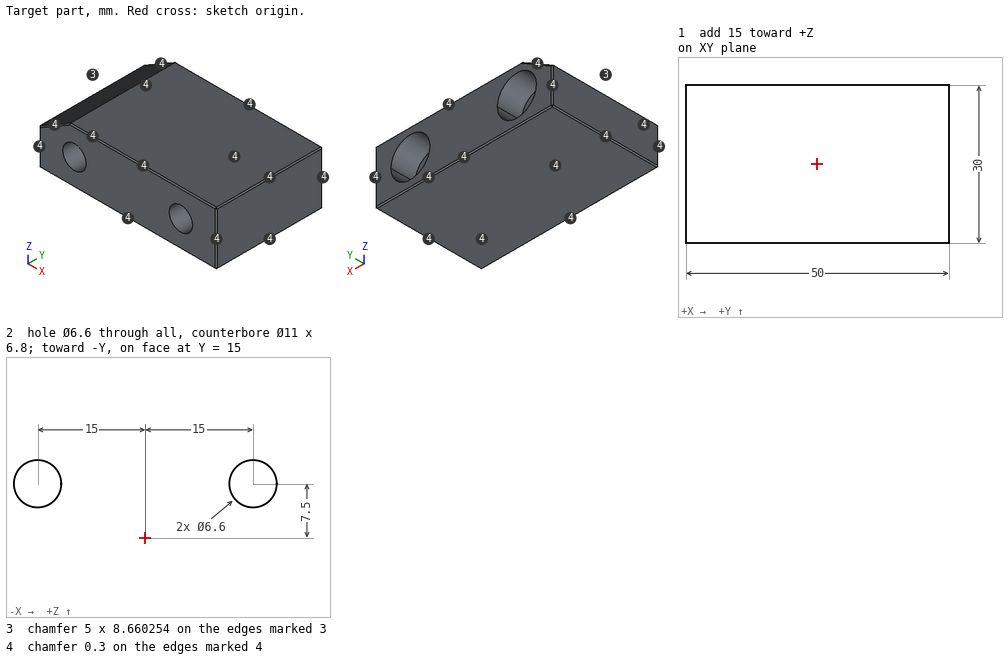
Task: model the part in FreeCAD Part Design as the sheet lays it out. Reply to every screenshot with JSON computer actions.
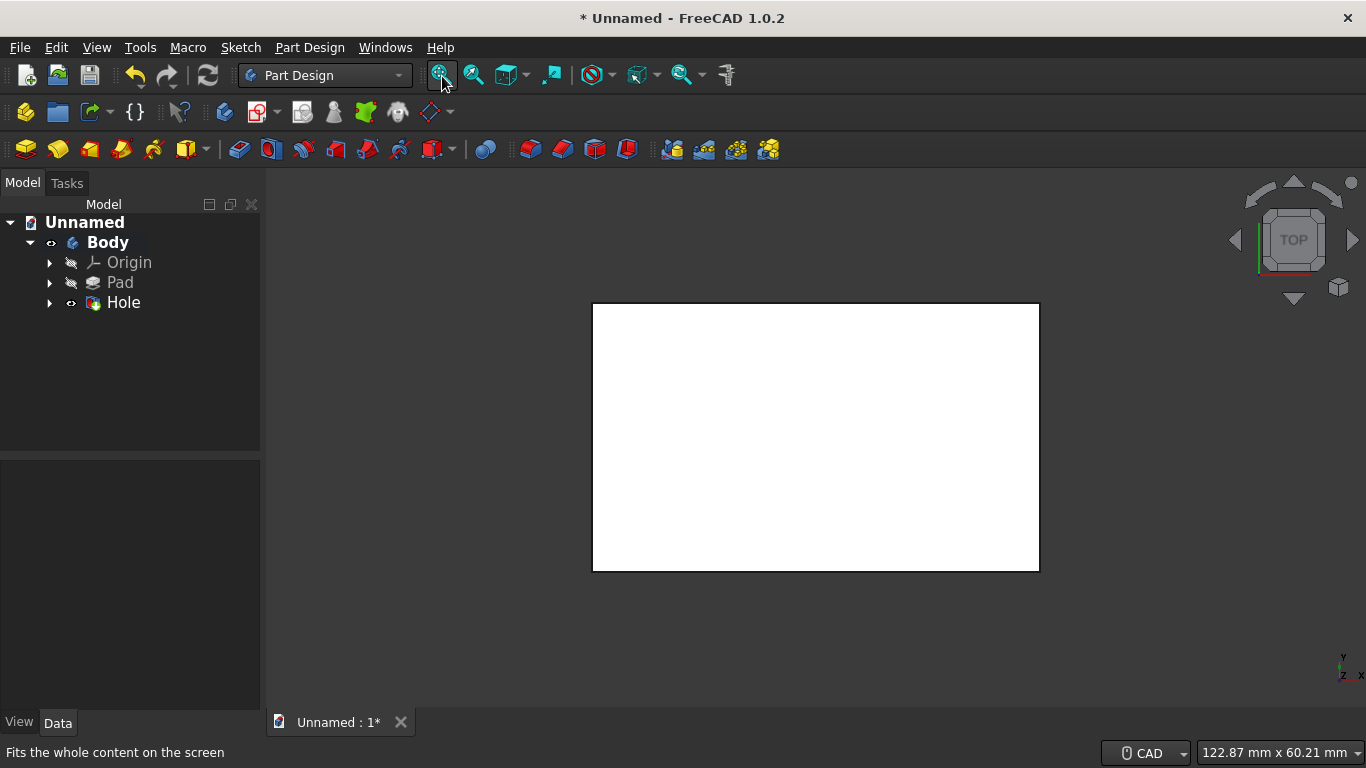
{"action": "left_click", "coordinate": [592, 437]}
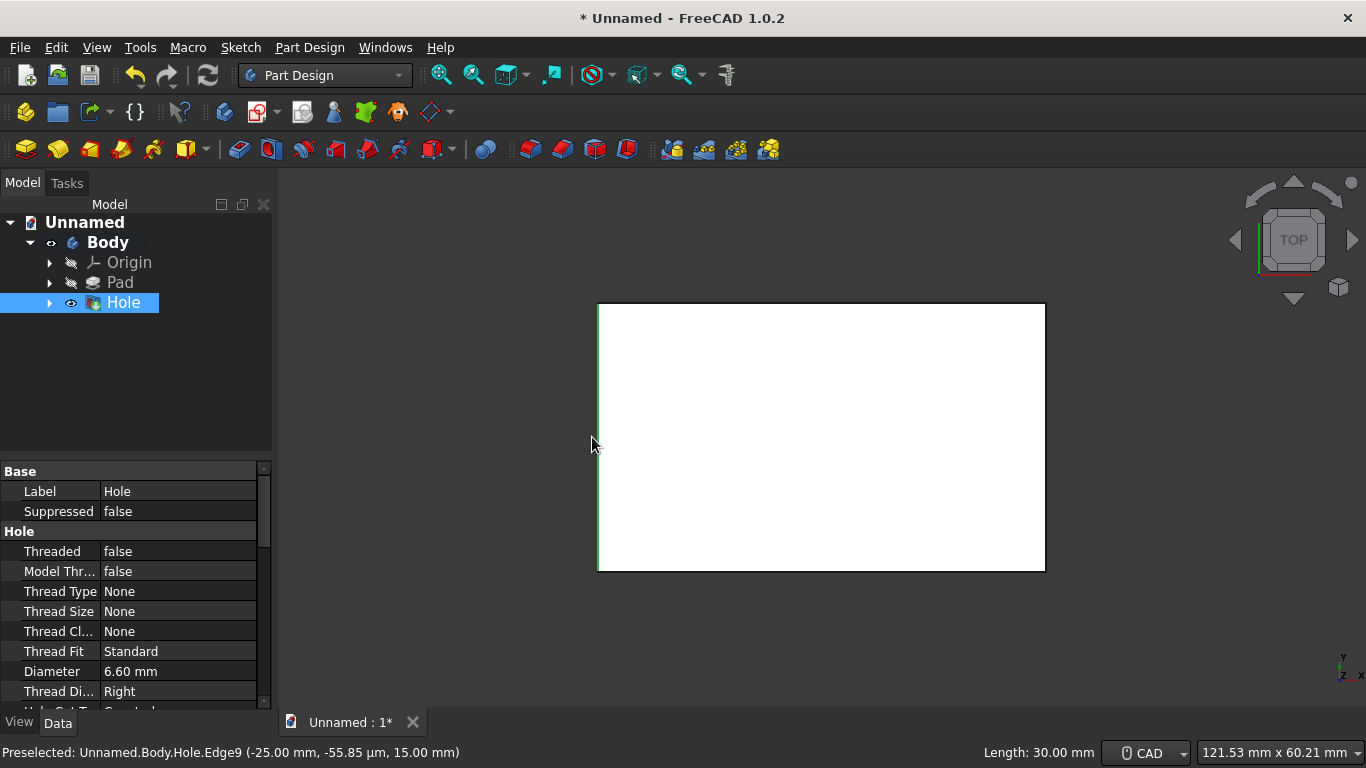
{"action": "left_click", "coordinate": [564, 150]}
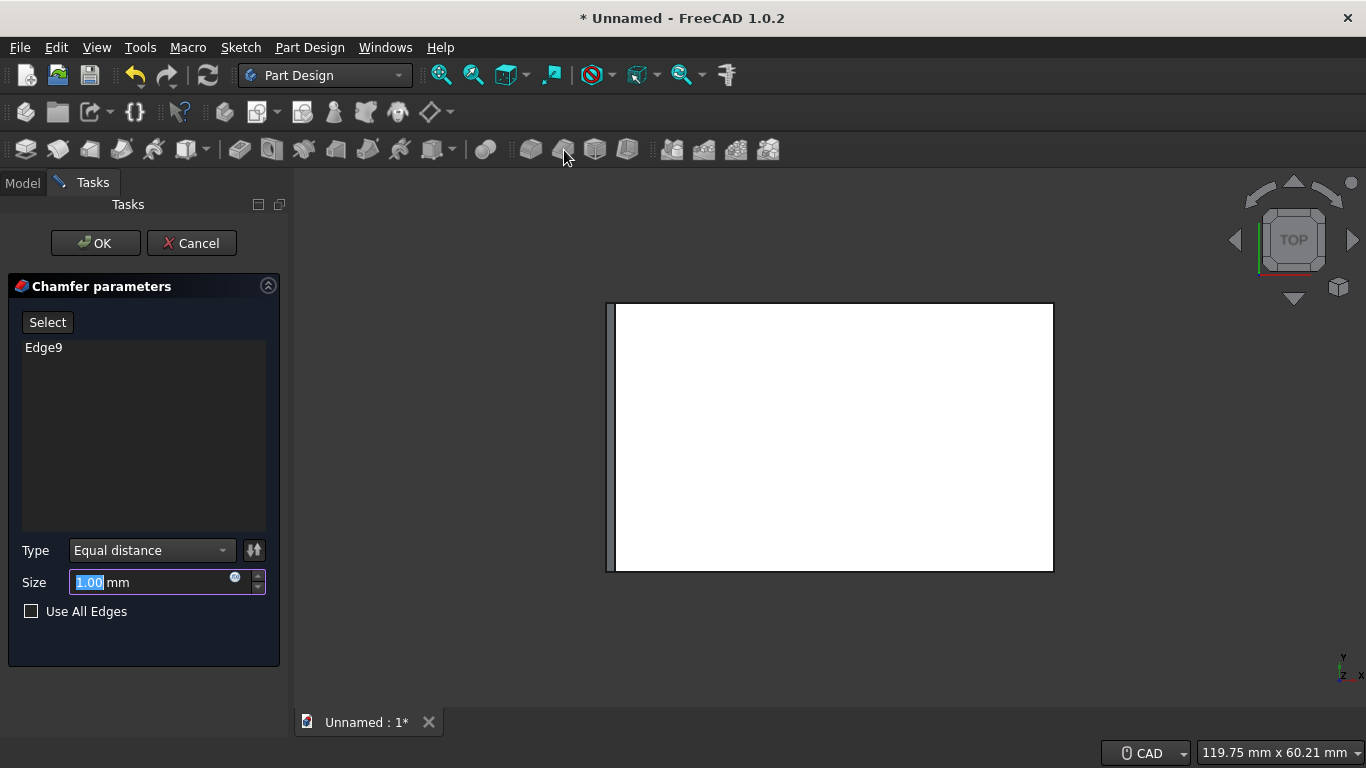
{"action": "type", "text": "5"}
{"action": "key", "text": "Tab"}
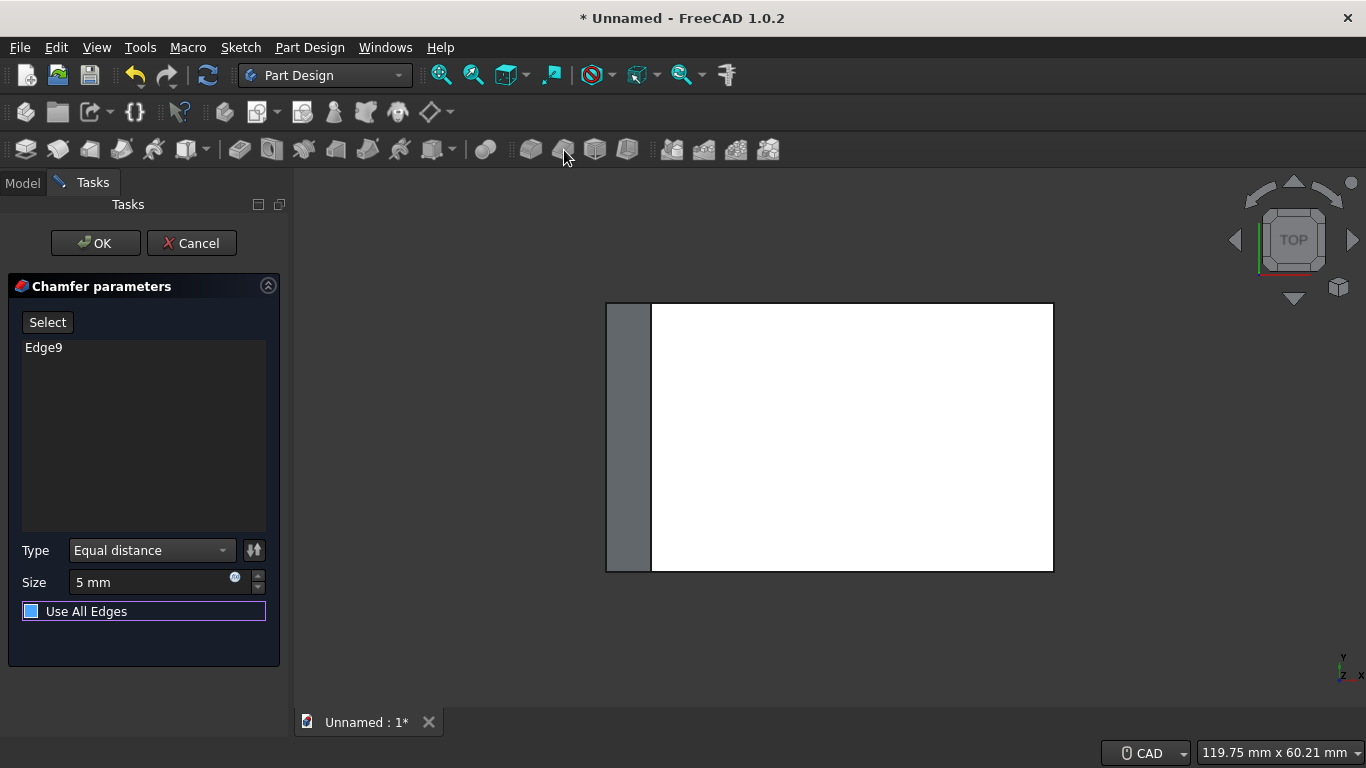
{"action": "left_click", "coordinate": [153, 550]}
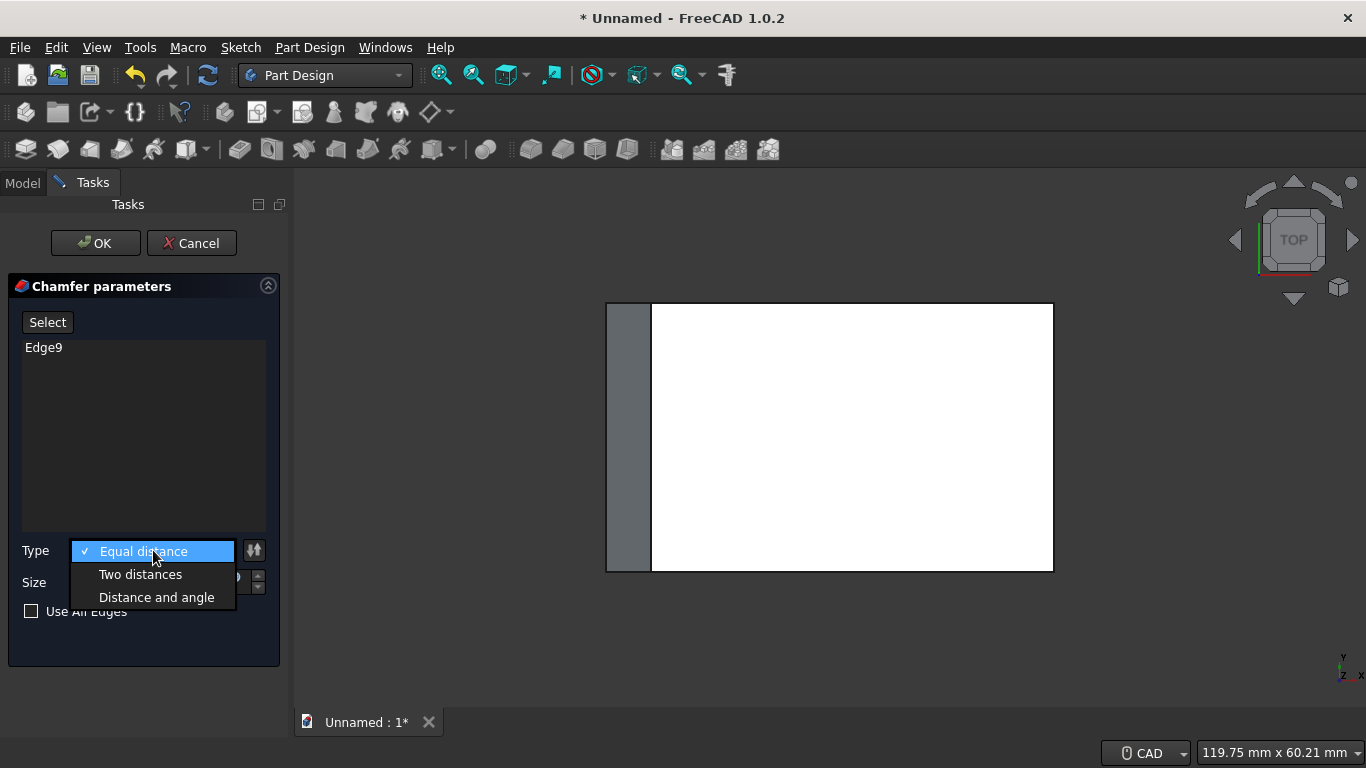
{"action": "left_click", "coordinate": [152, 574]}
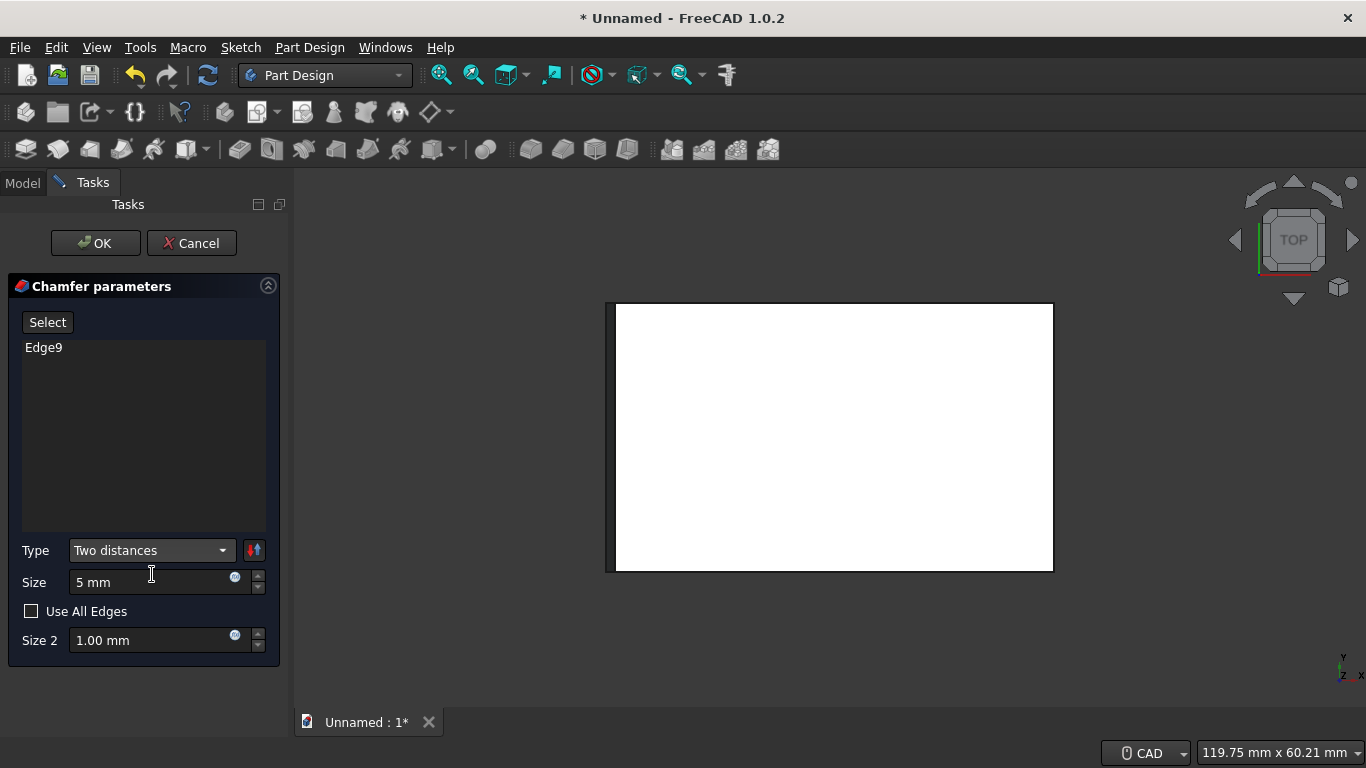
{"action": "triple_click", "coordinate": [160, 640]}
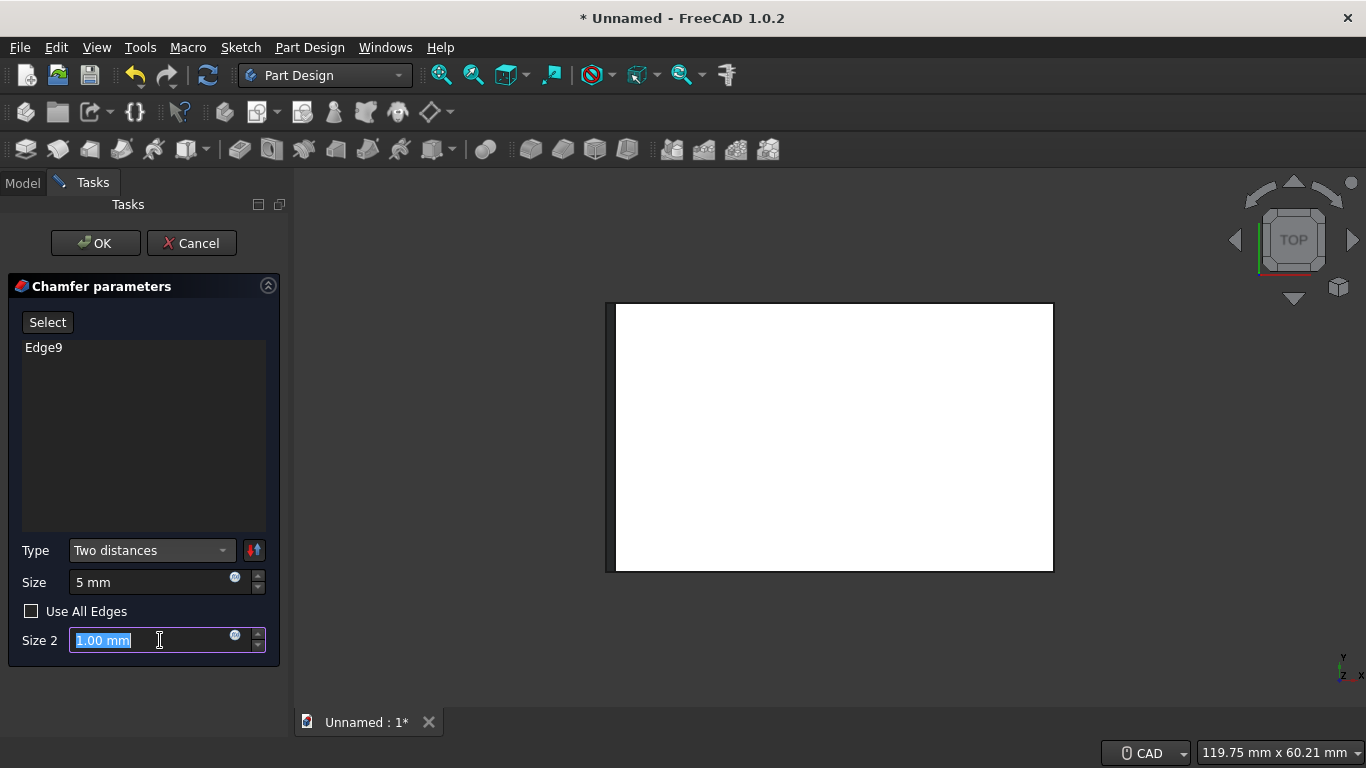
{"action": "type", "text": "8.660254"}
{"action": "key", "text": "Tab"}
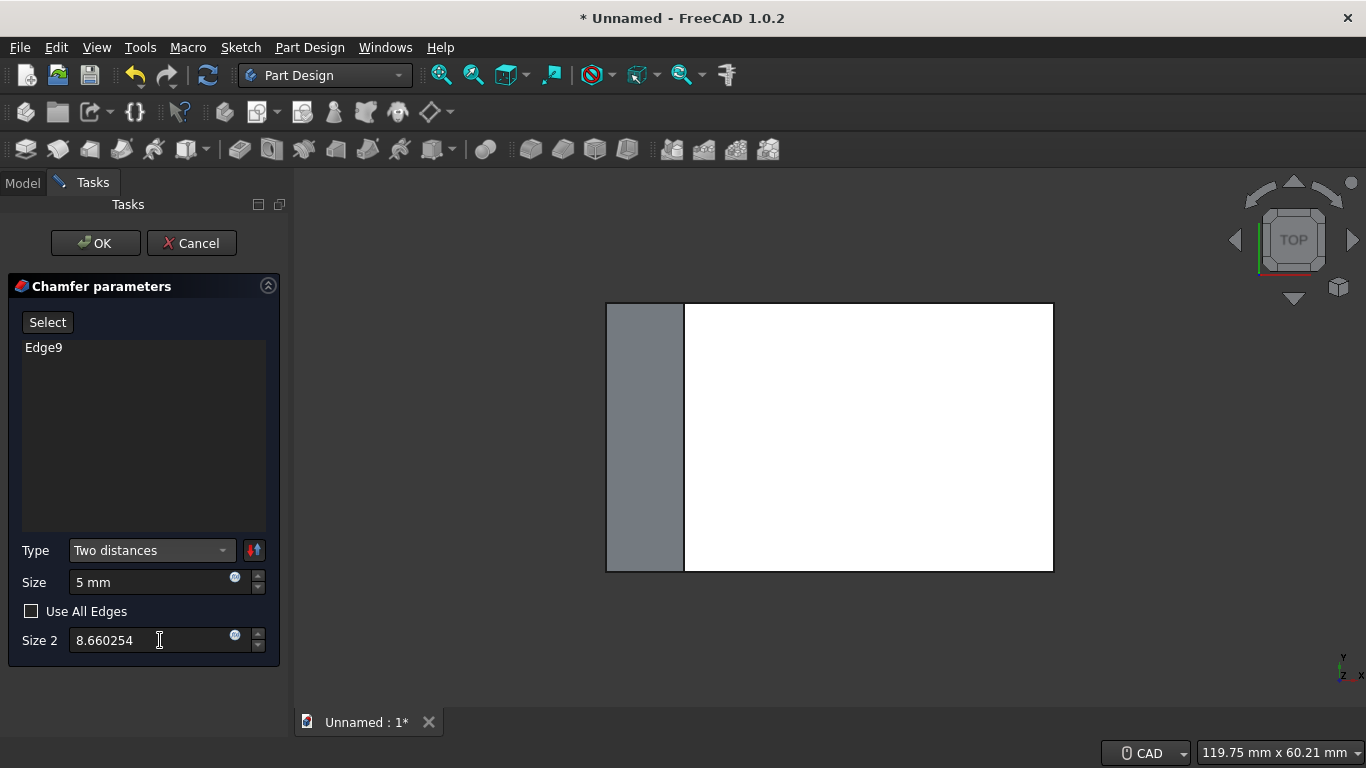
{"action": "left_click", "coordinate": [96, 243]}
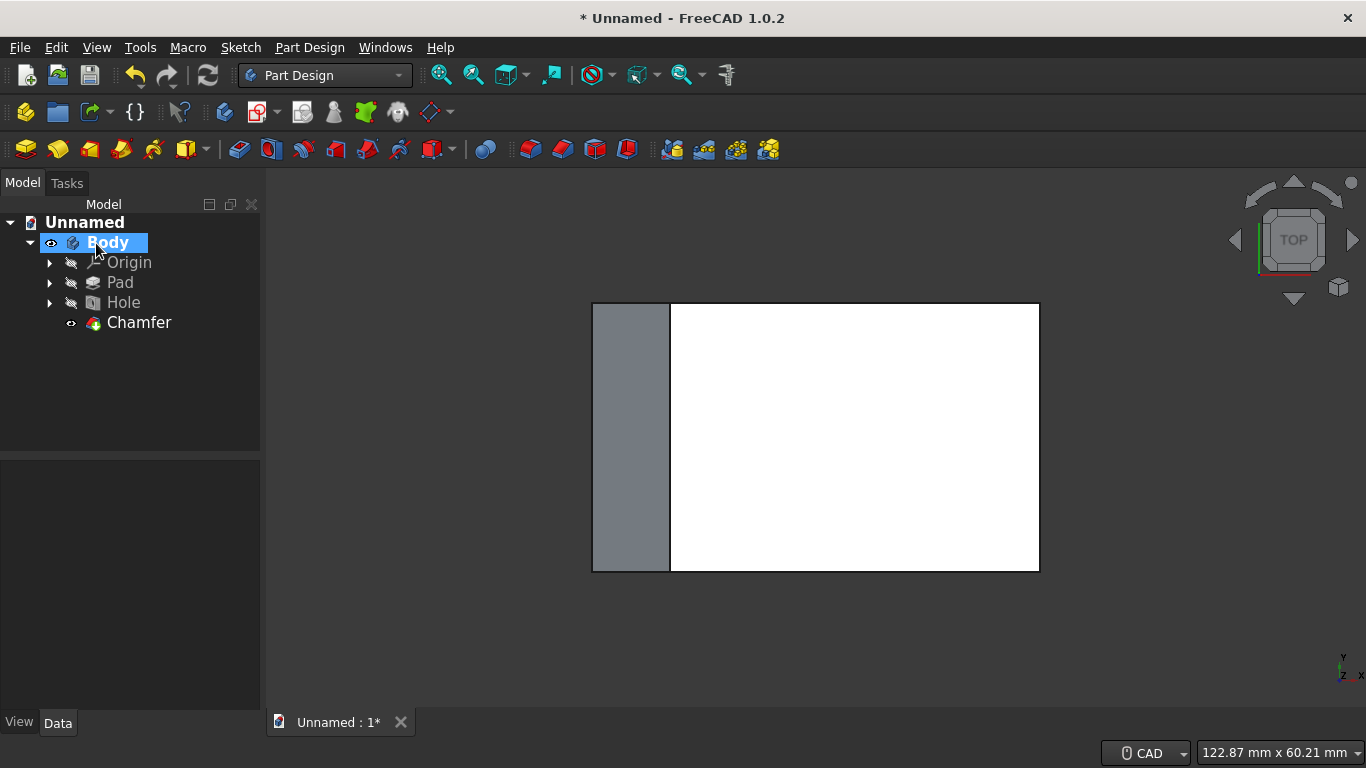
{"action": "left_click", "coordinate": [855, 571]}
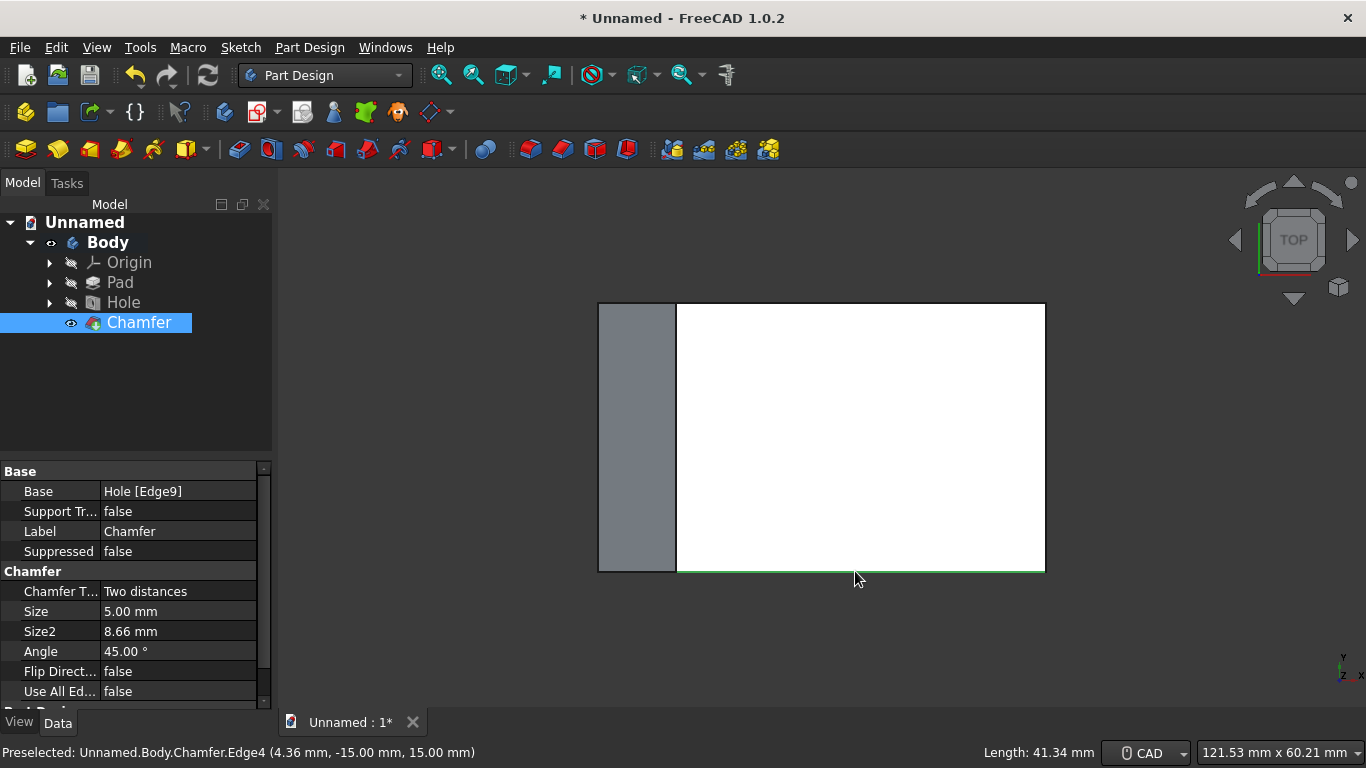
{"action": "left_click", "coordinate": [637, 571], "text": "ctrl"}